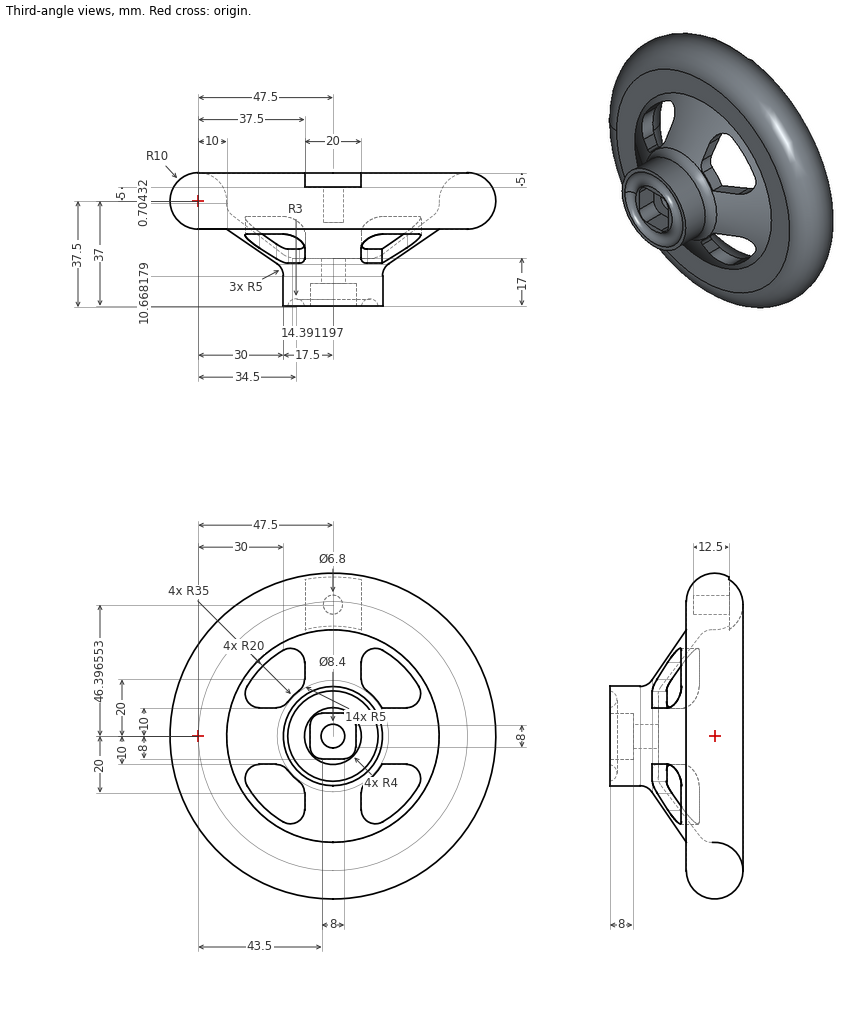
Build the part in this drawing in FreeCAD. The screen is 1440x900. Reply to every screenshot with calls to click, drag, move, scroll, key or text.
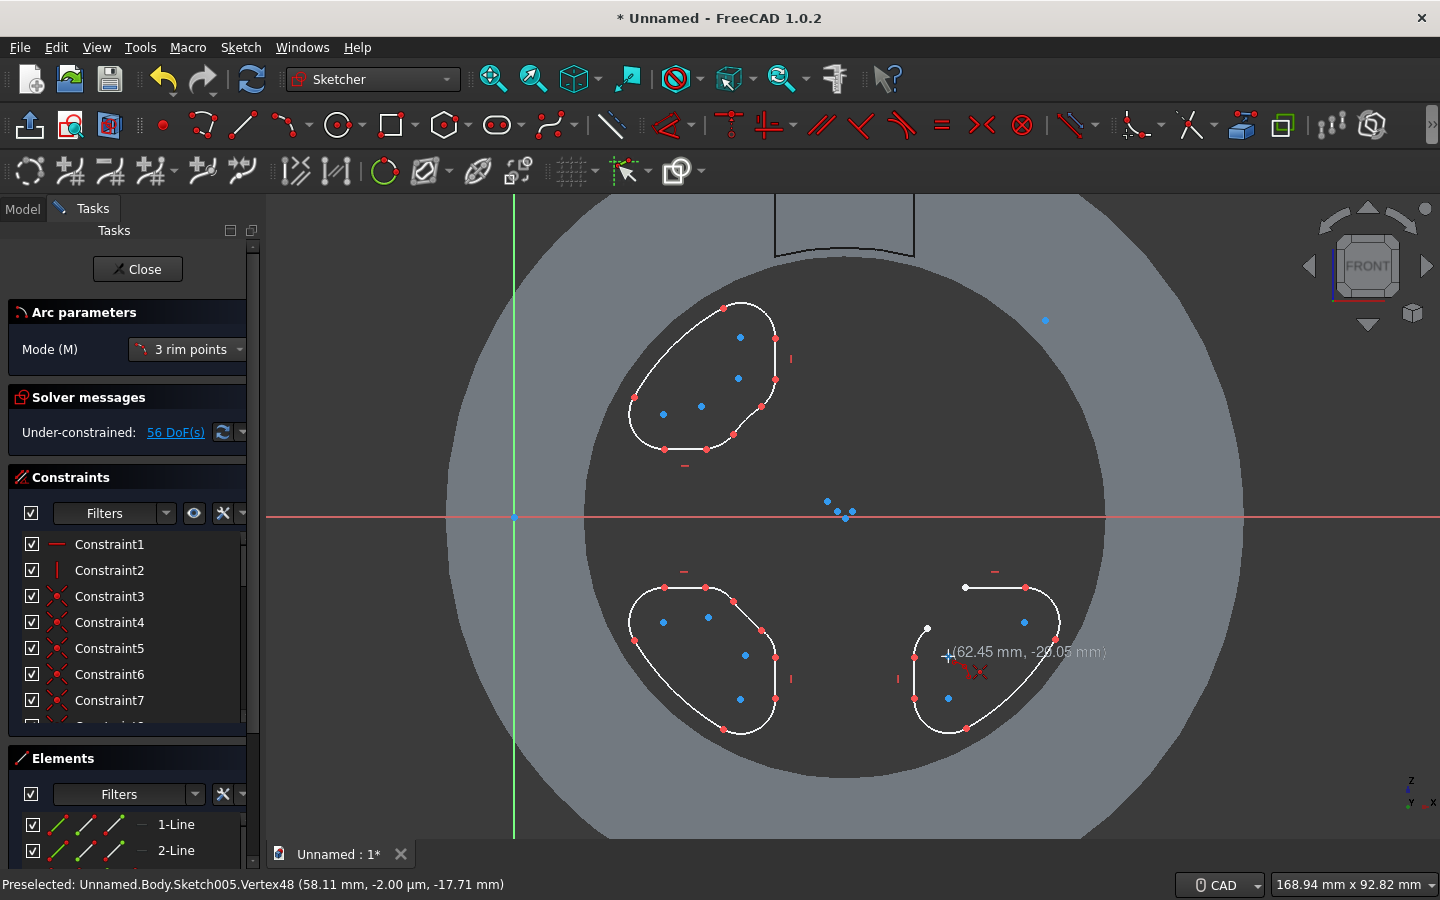
click(928, 629)
click(965, 588)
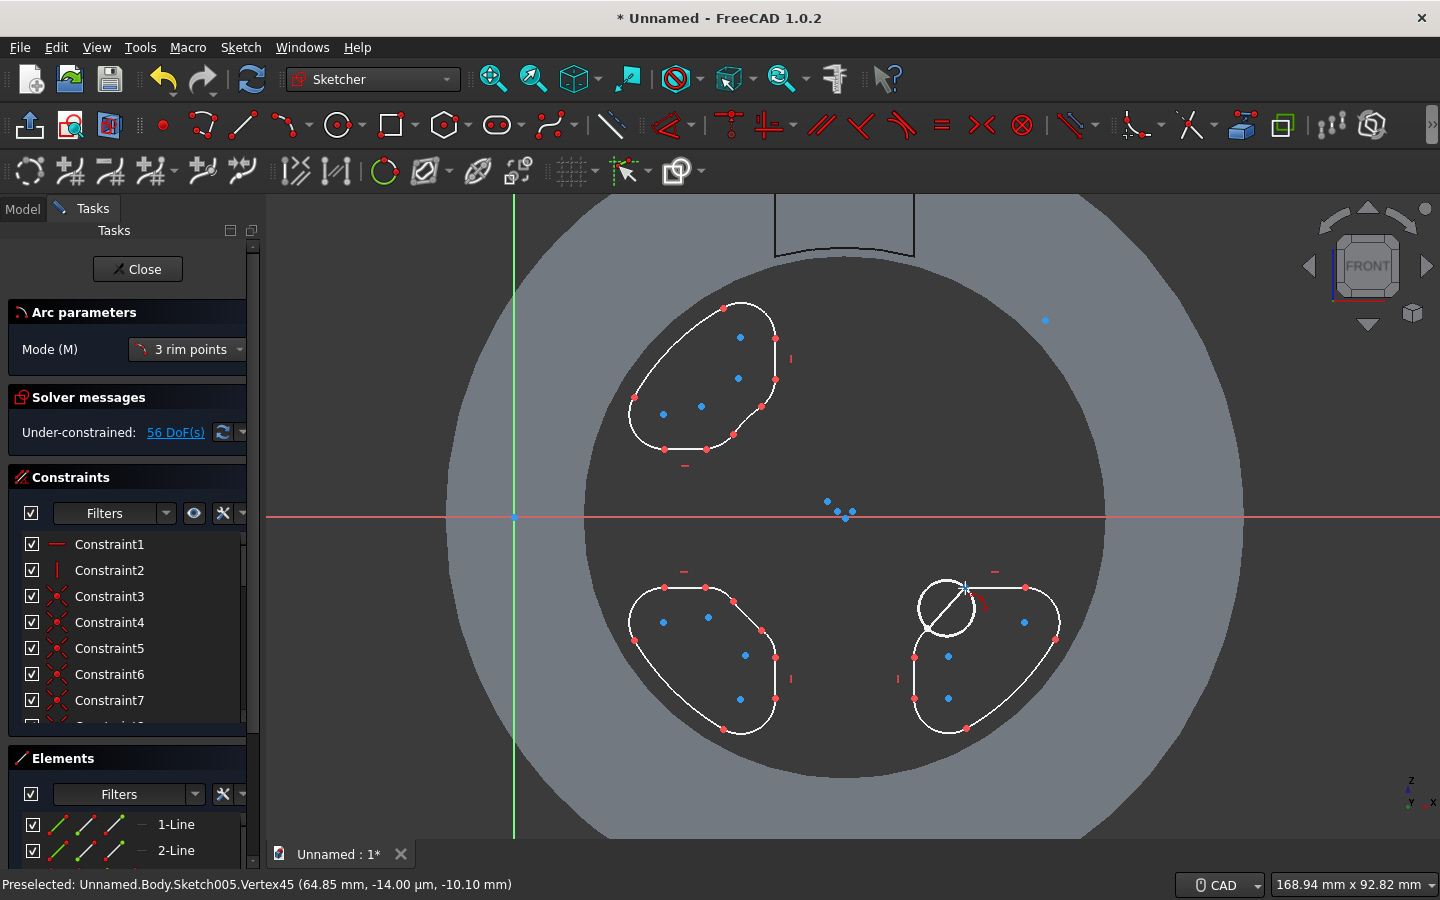
scroll(949, 610, up, 9)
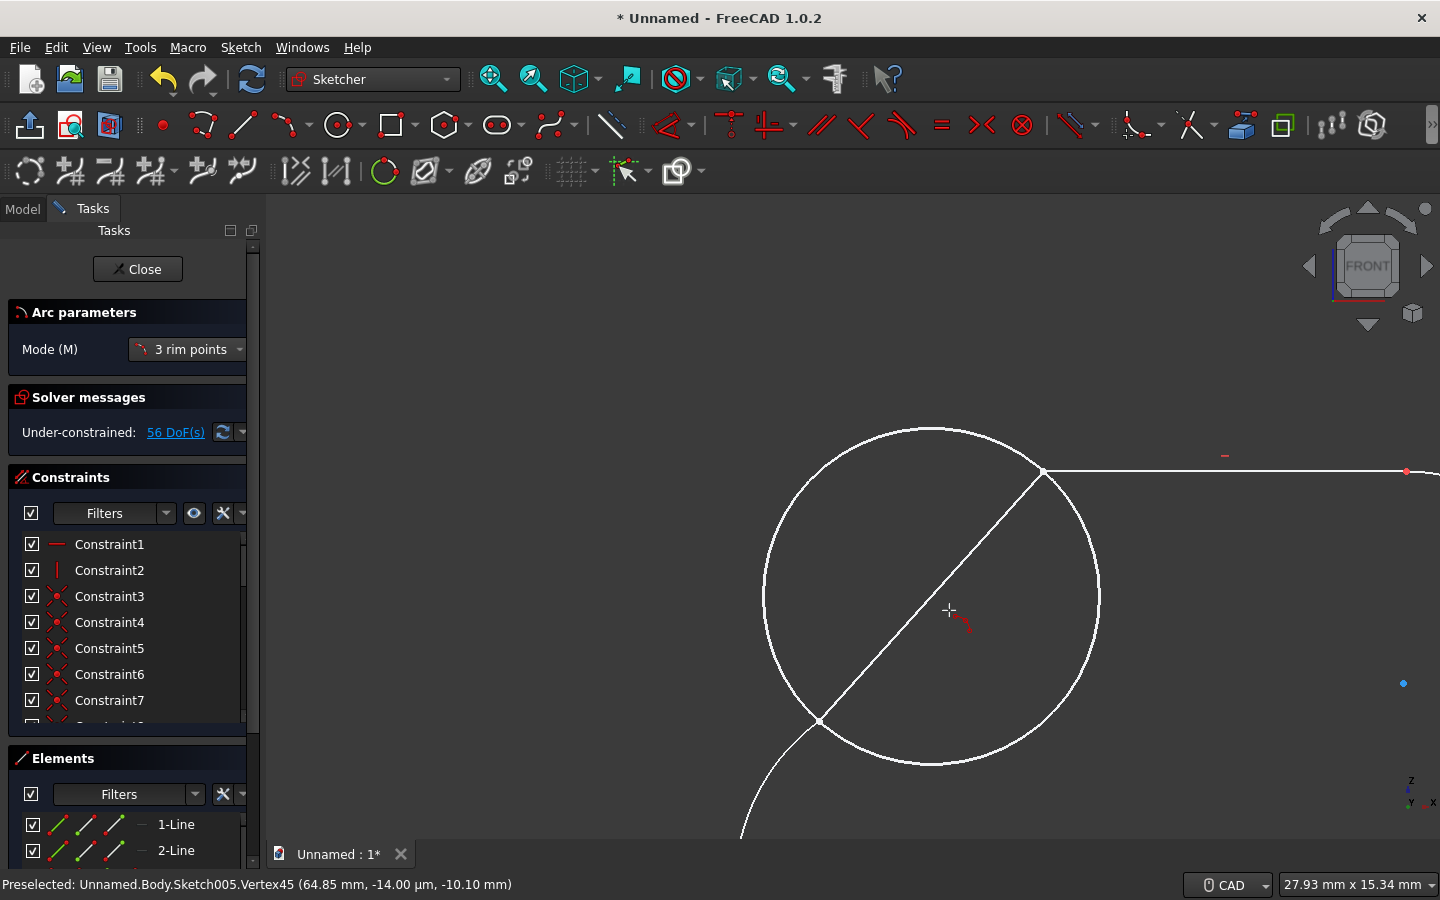
click(943, 605)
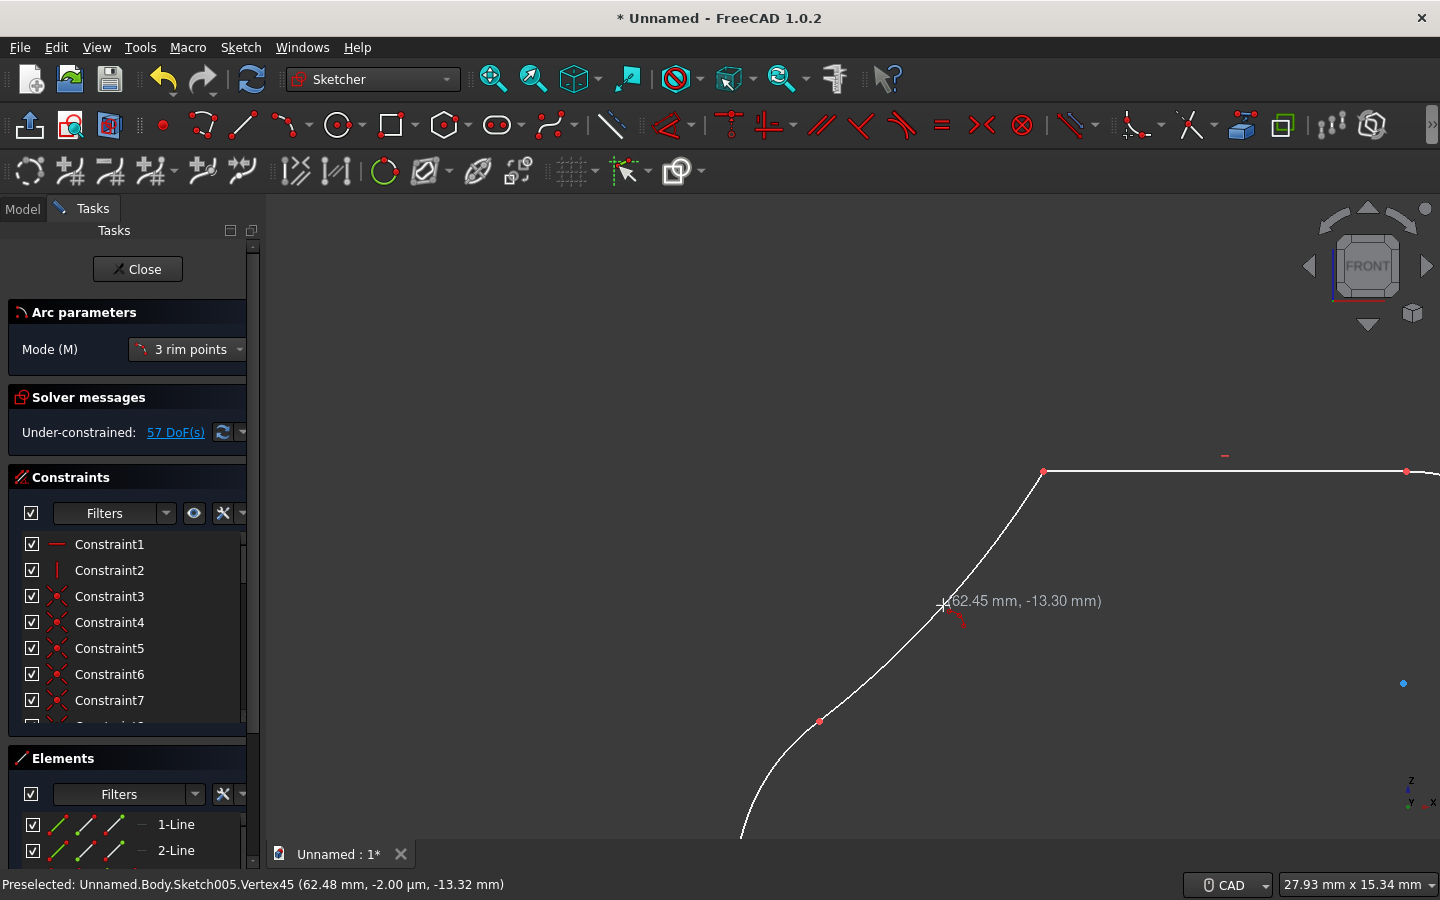
click(244, 126)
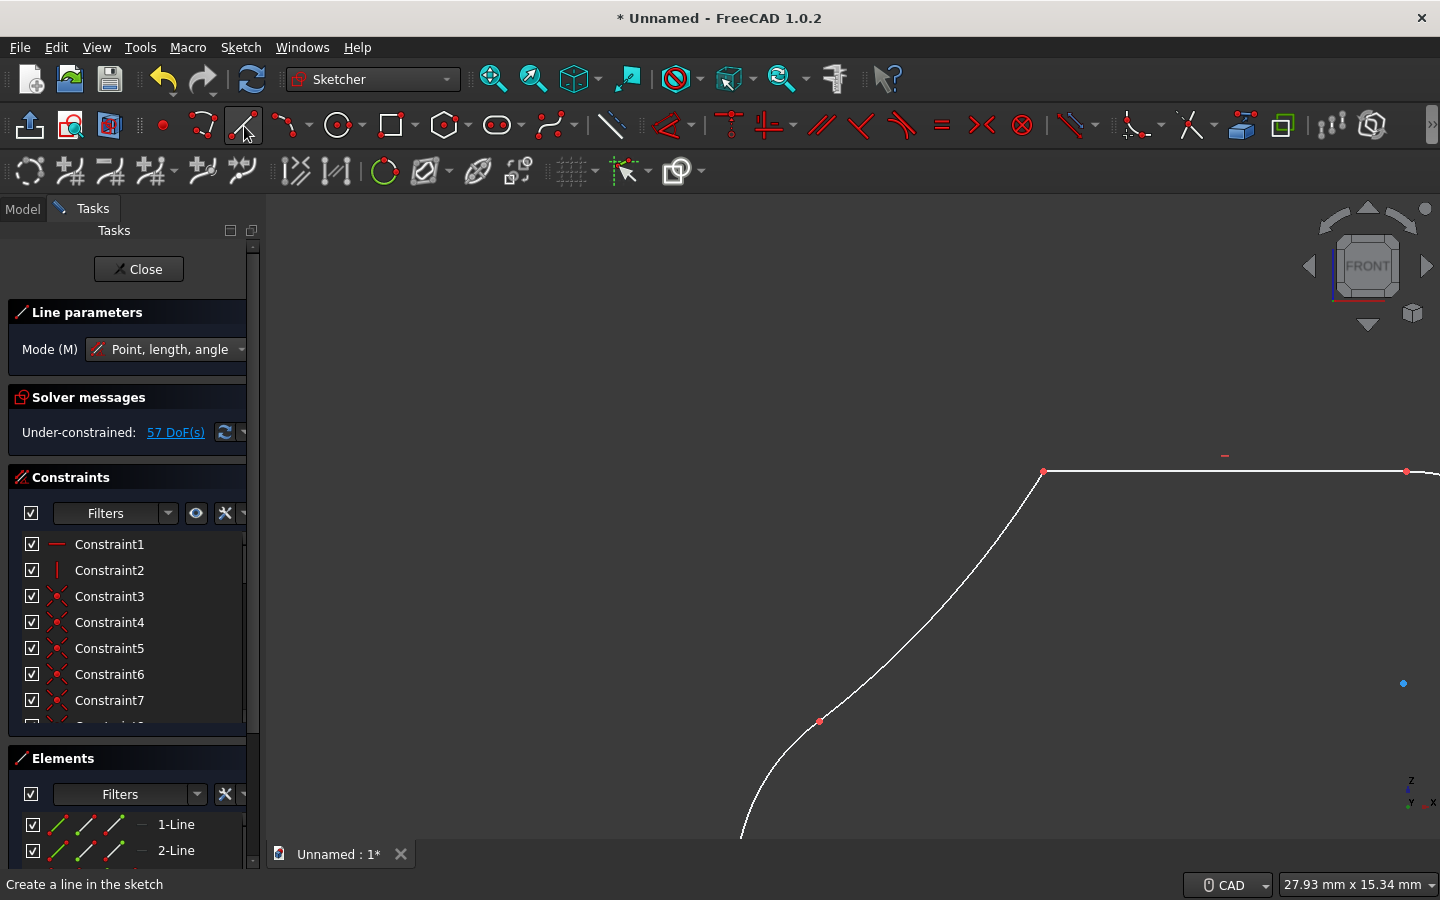
scroll(949, 610, down, 9)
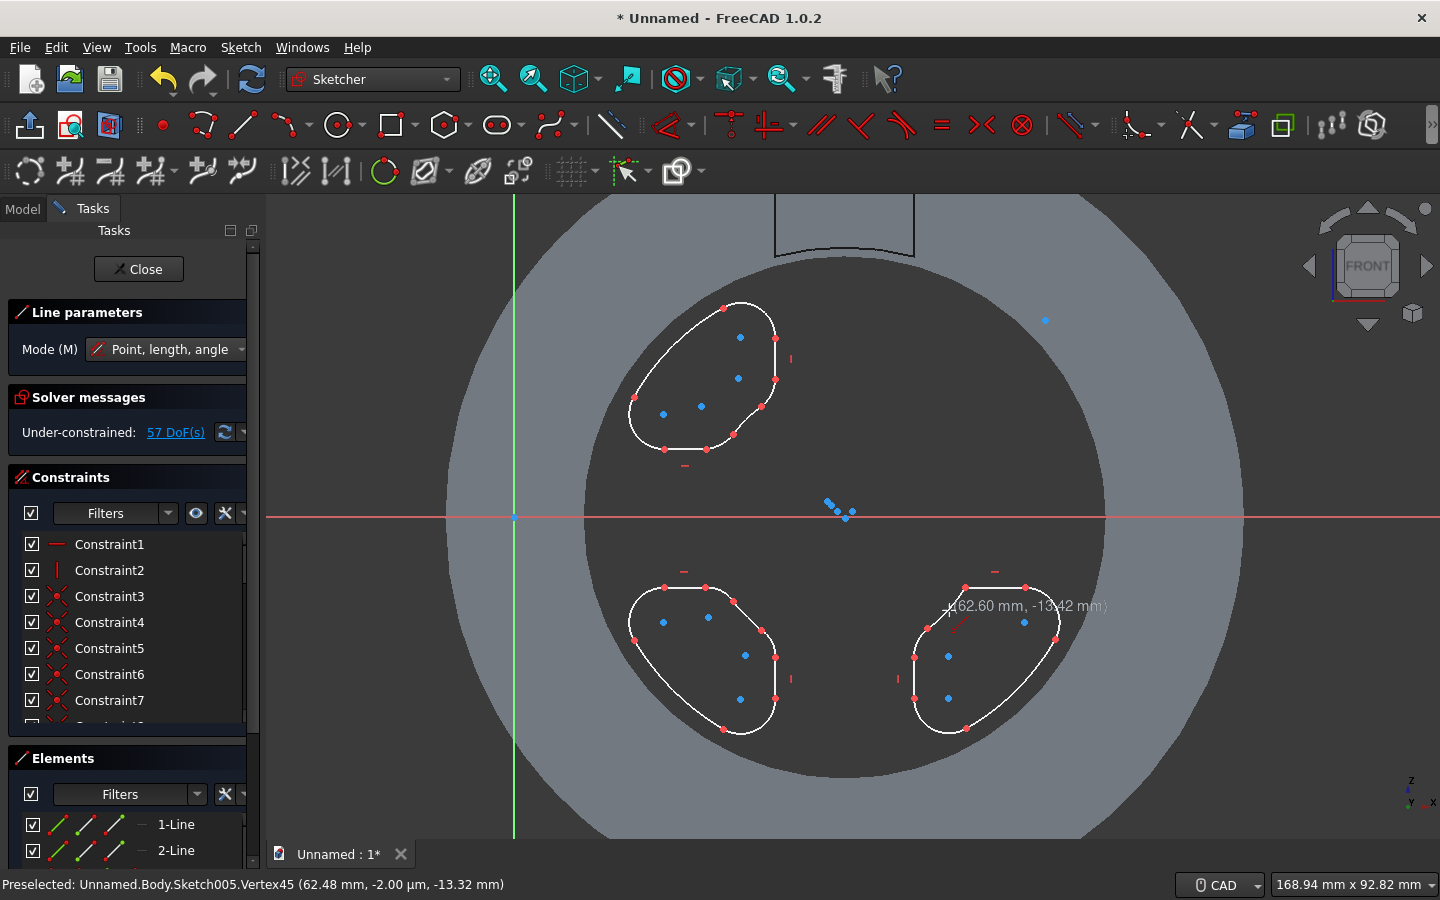
click(1025, 448)
click(965, 448)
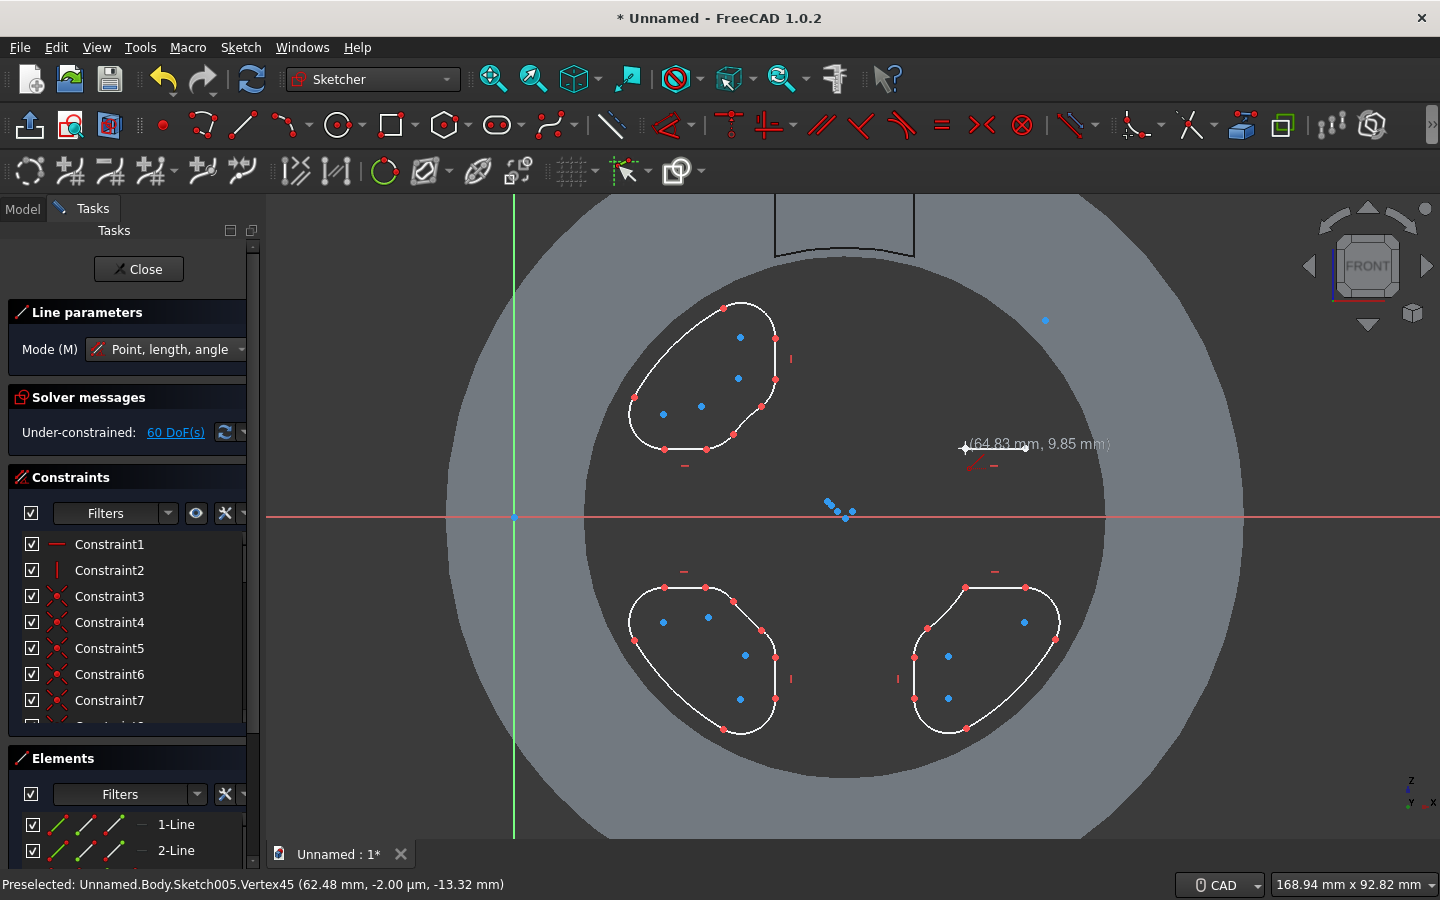
click(914, 378)
click(914, 337)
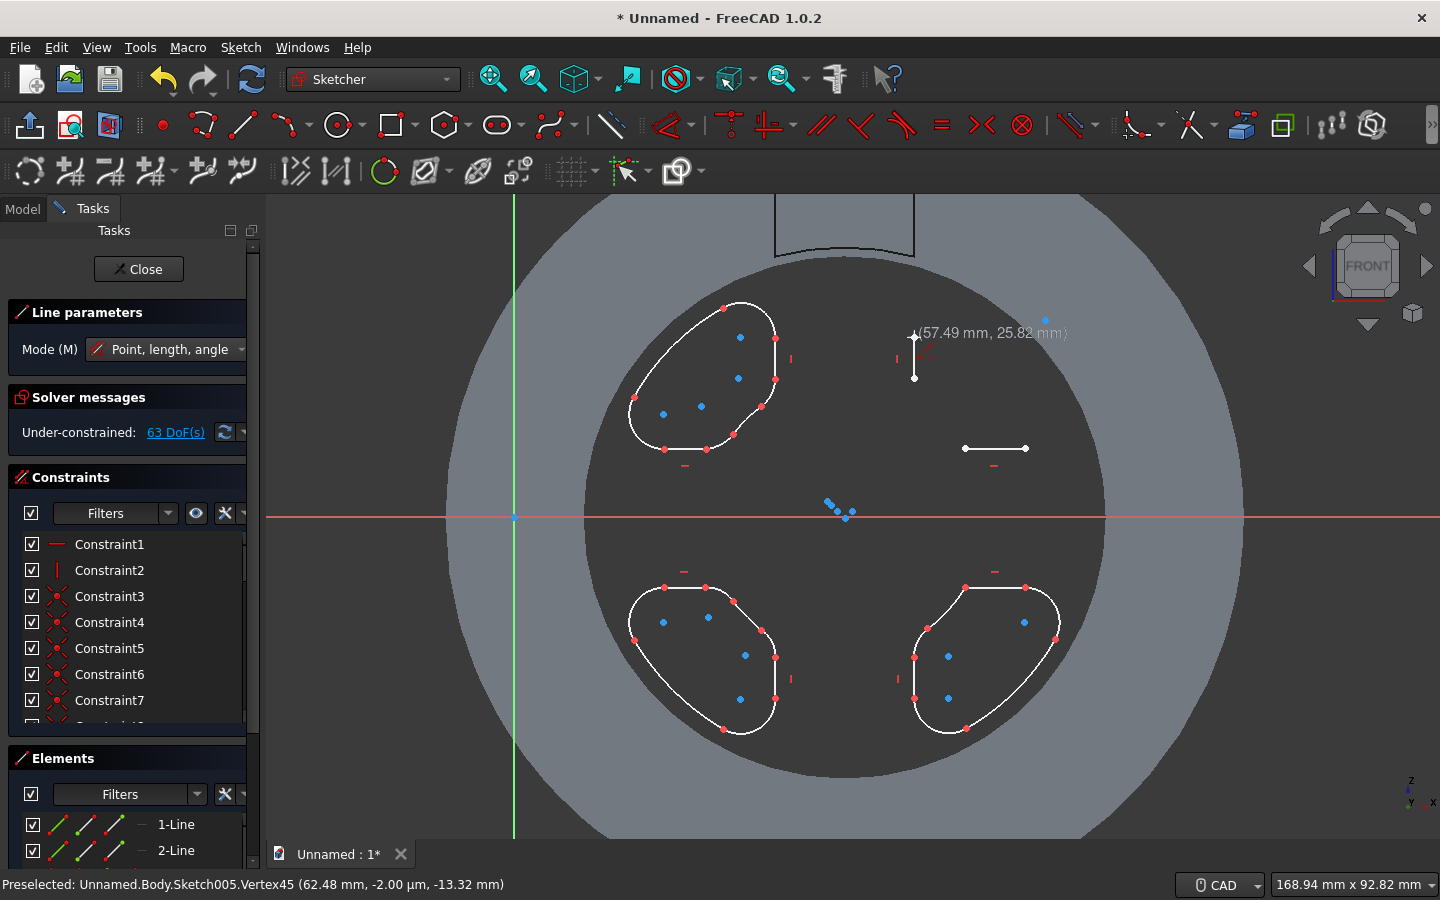
click(284, 126)